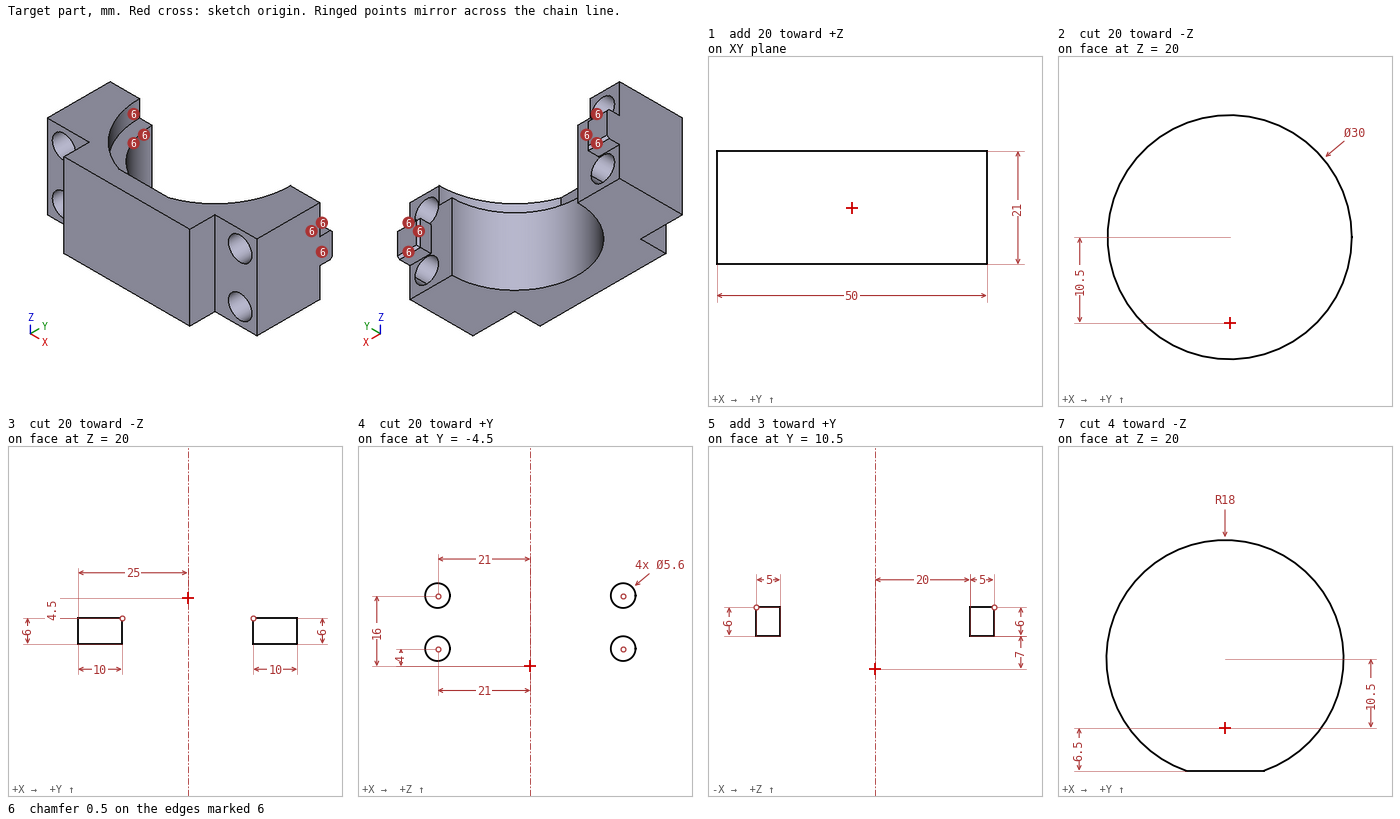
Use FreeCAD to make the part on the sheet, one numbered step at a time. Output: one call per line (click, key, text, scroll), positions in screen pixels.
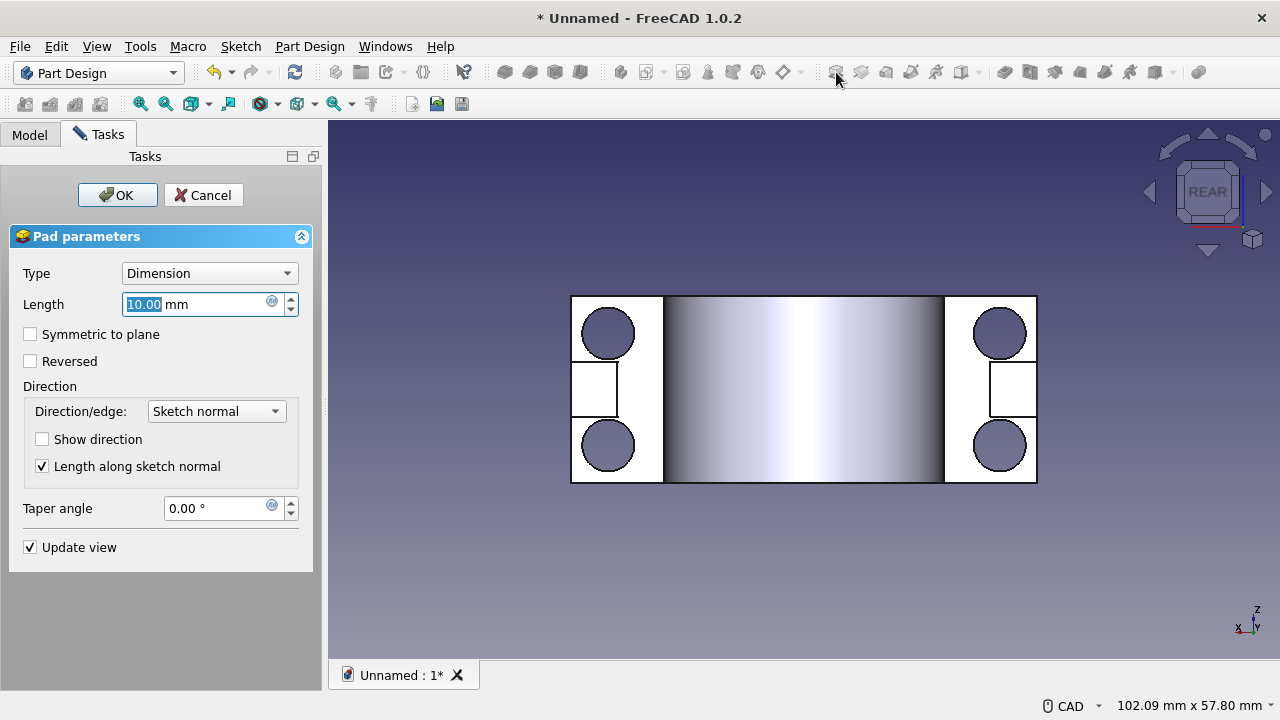
text(3)
key(Tab)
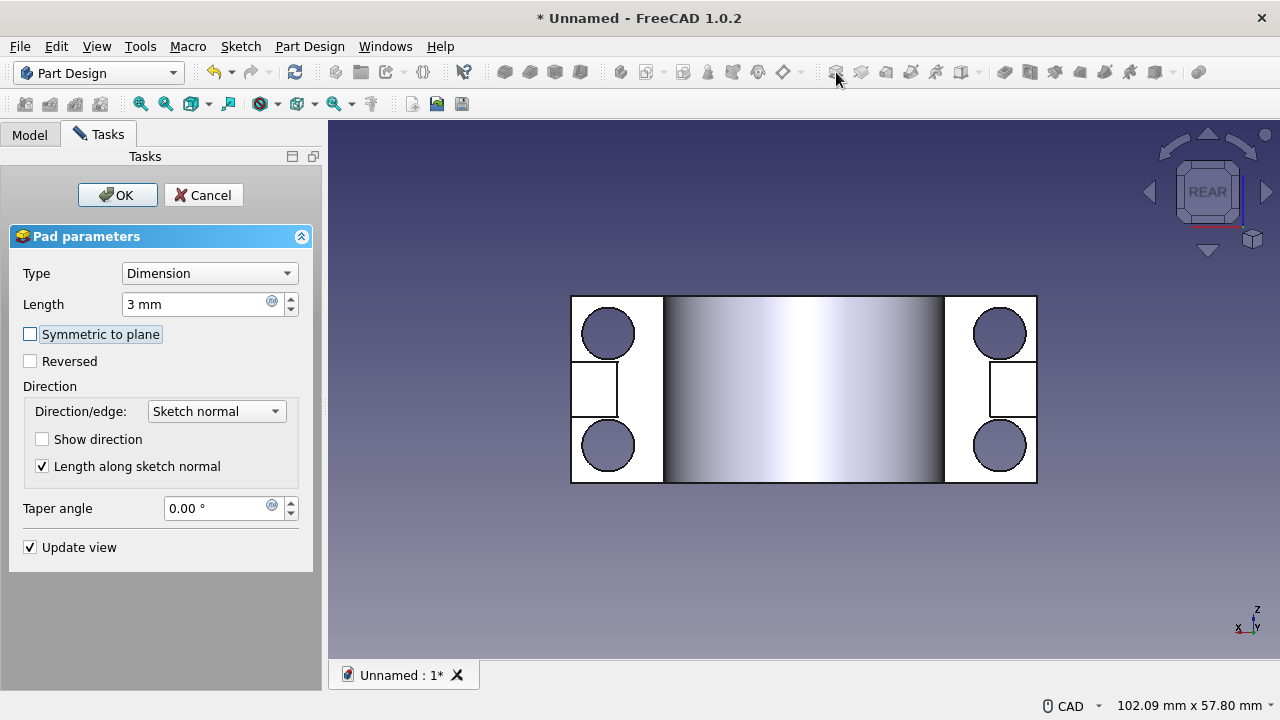
click(118, 195)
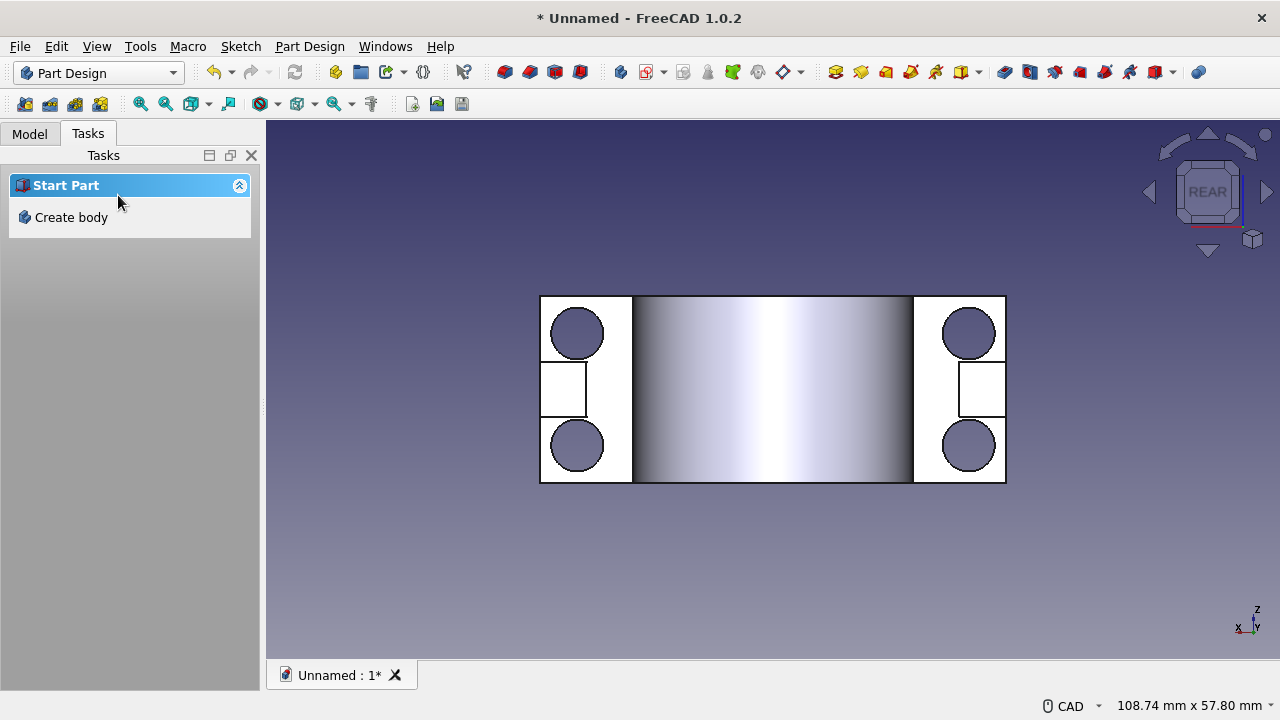
click(983, 361)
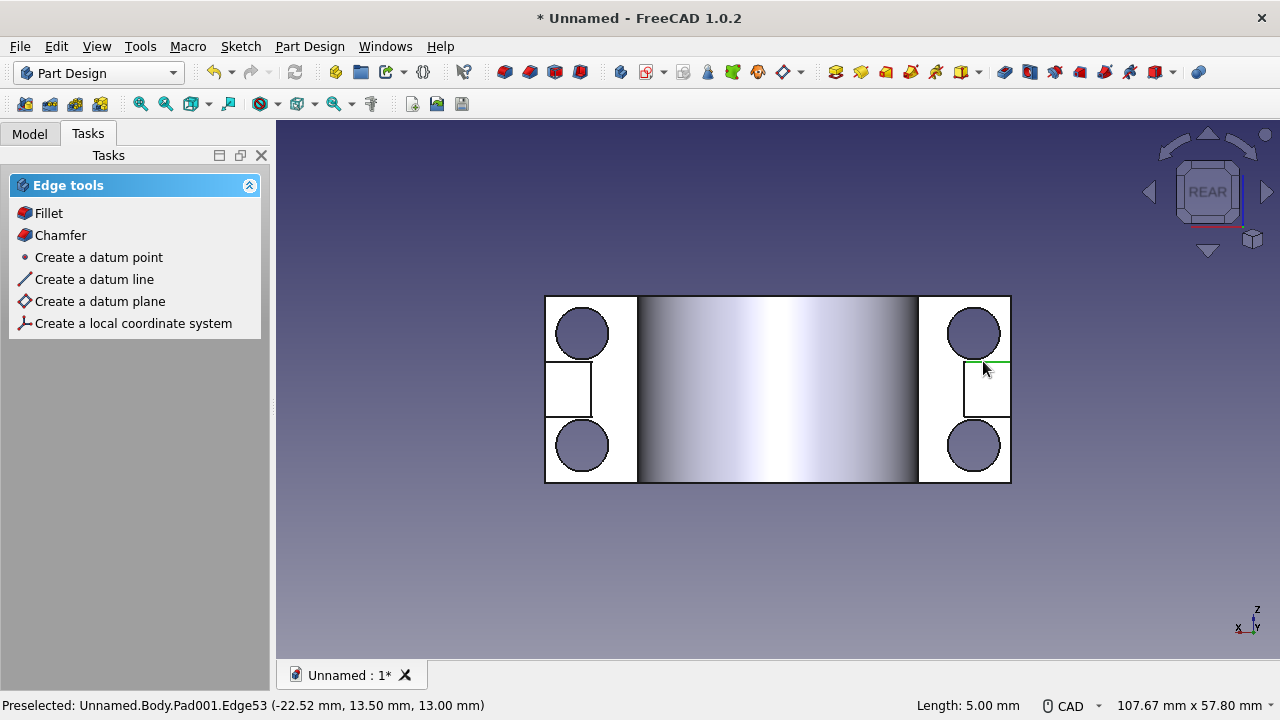
click(591, 389, ctrl)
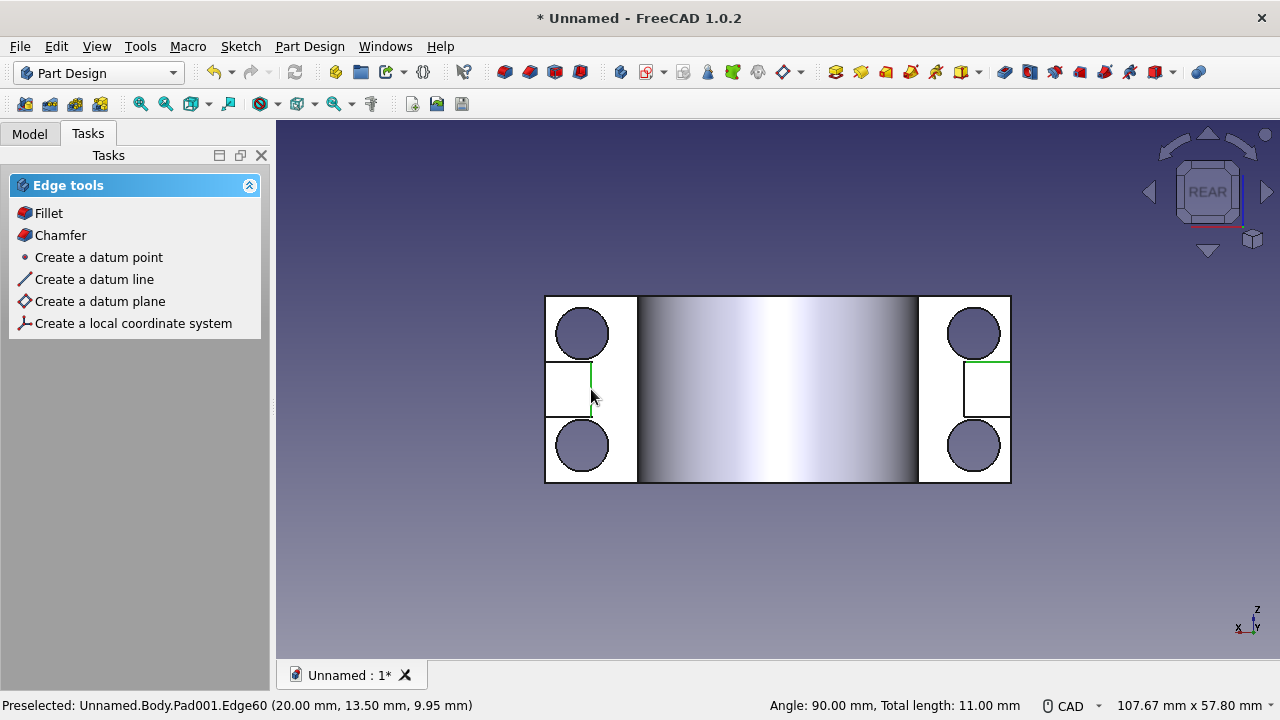
click(568, 361, ctrl)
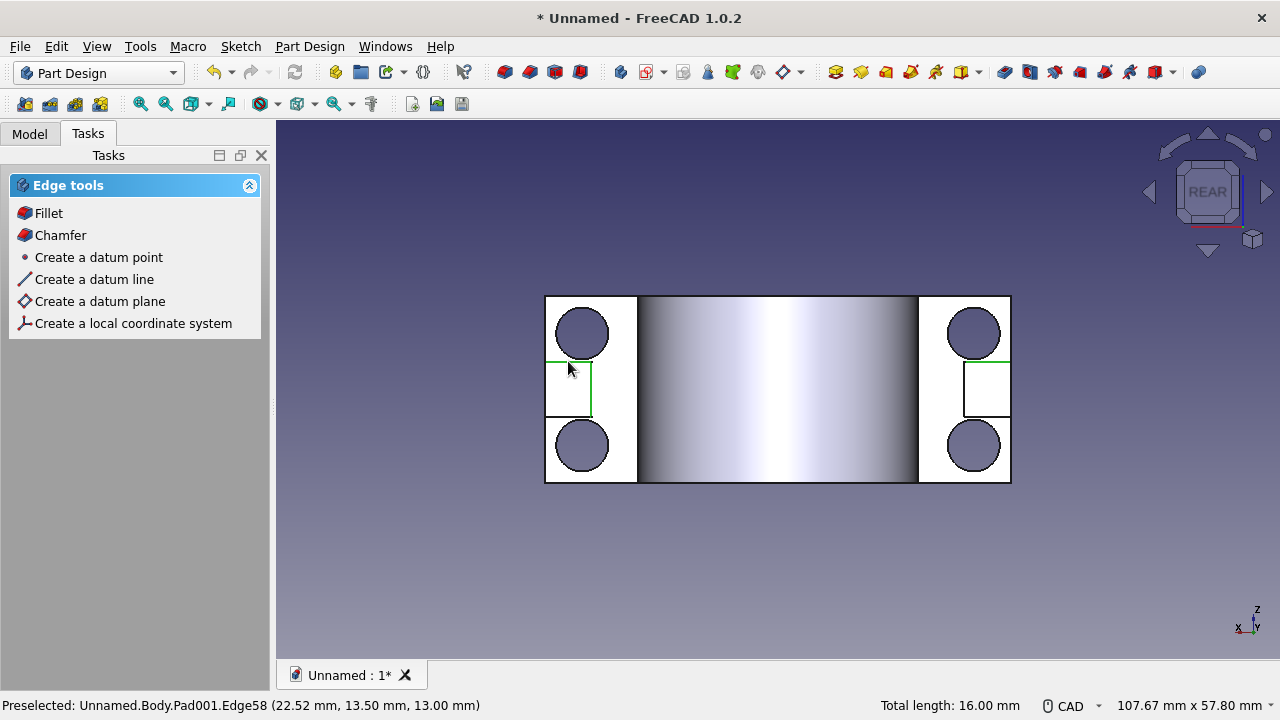
key(0)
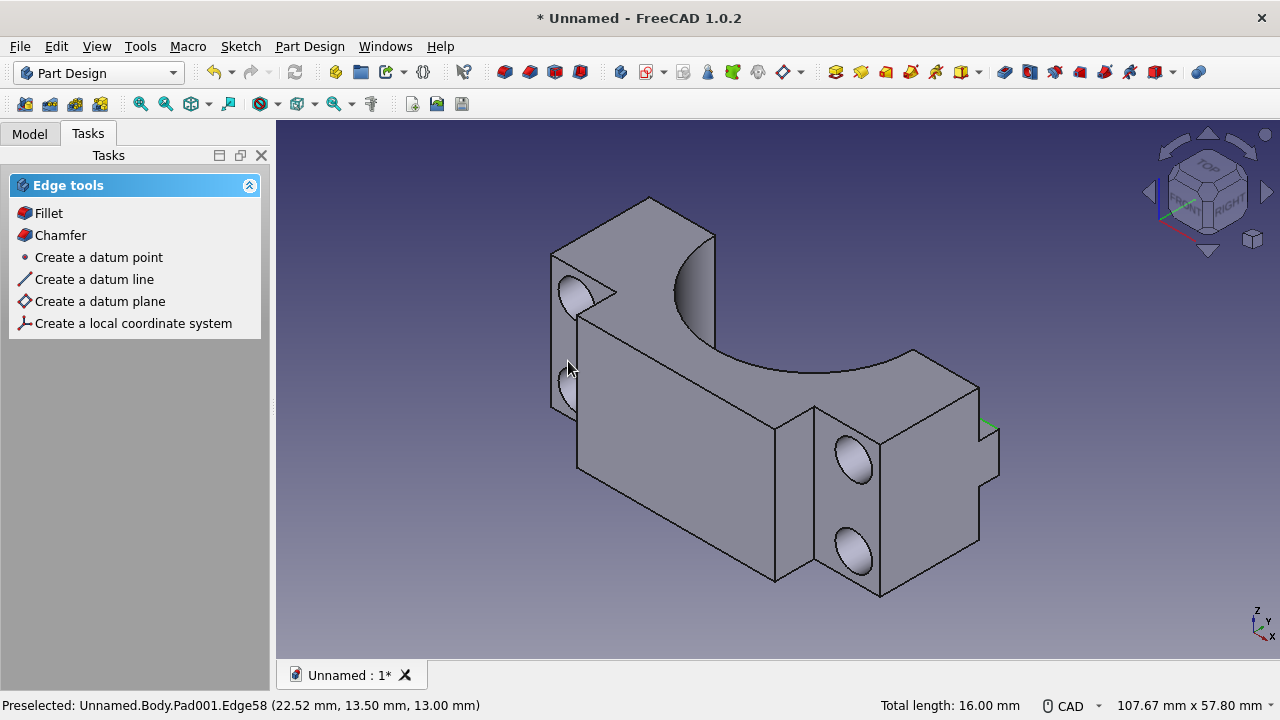
key(2)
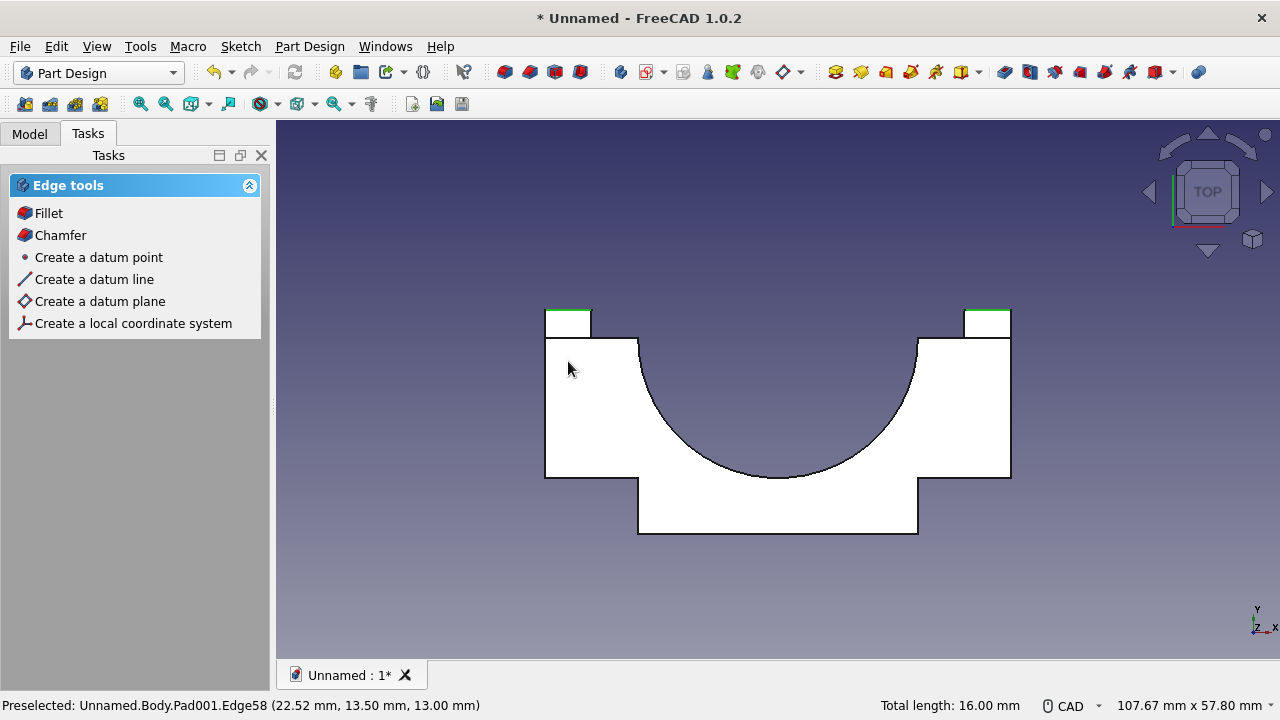
key(1)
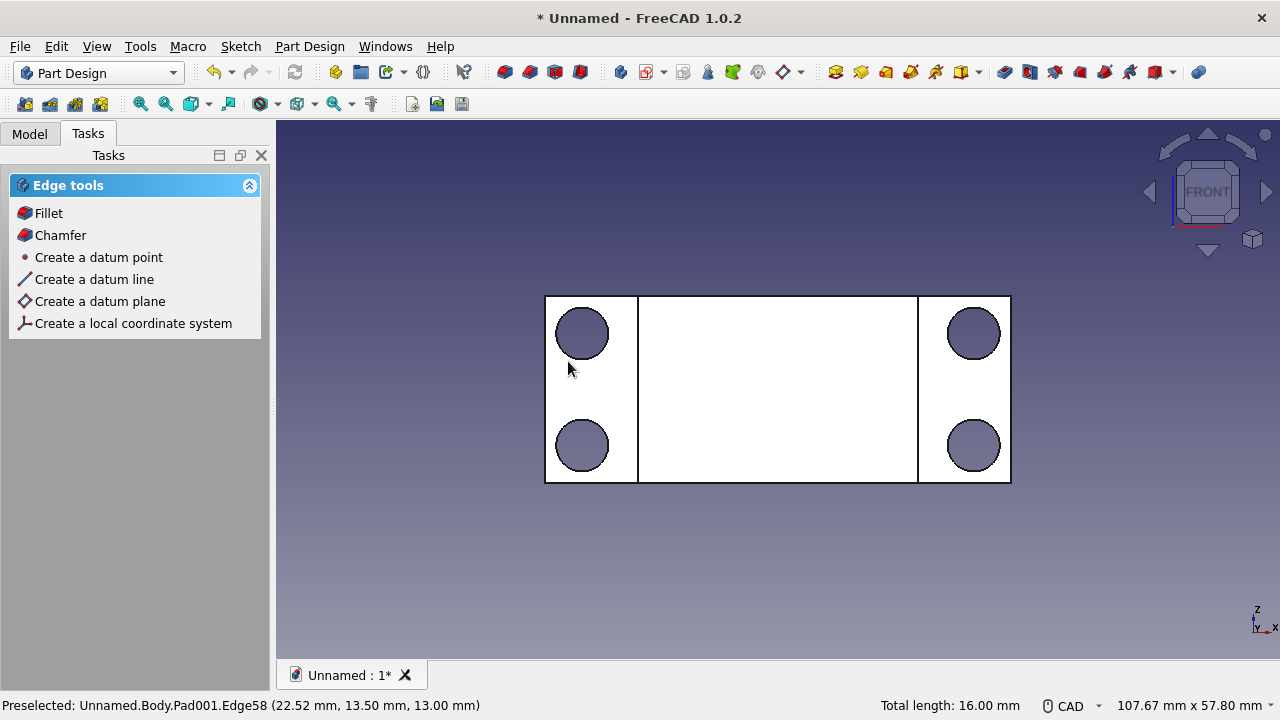
key(3)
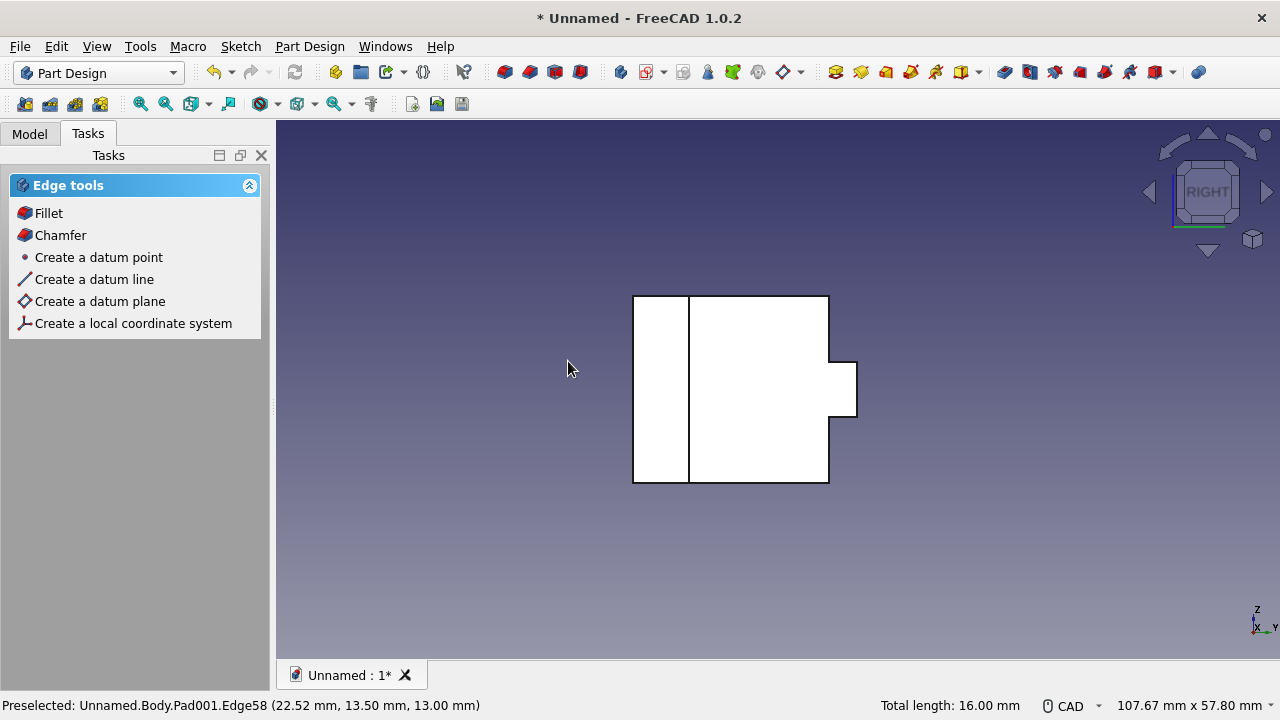
click(141, 104)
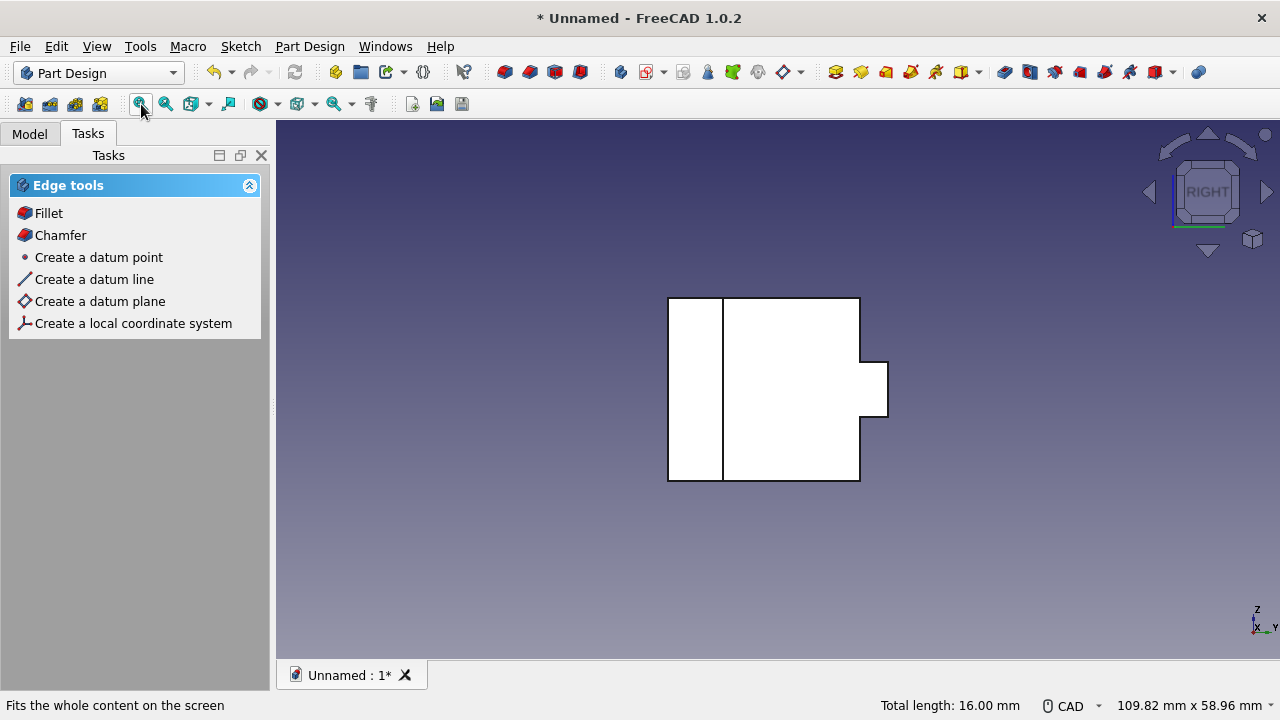
key(5)